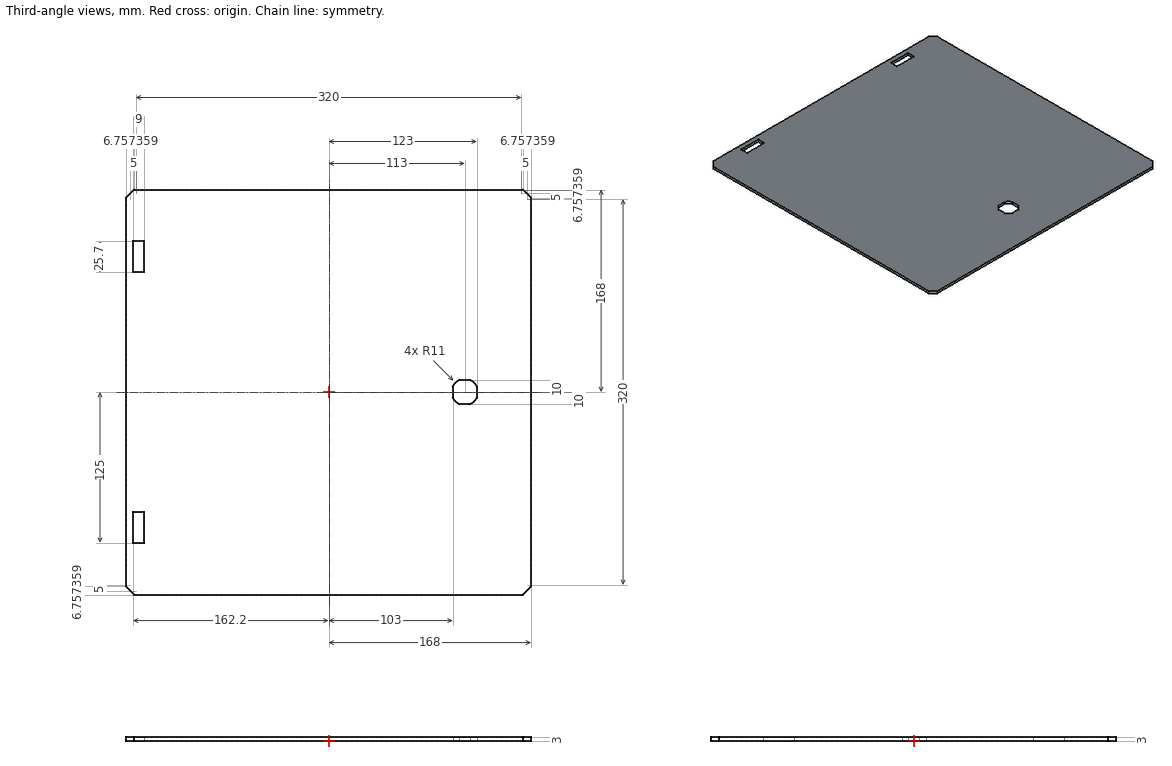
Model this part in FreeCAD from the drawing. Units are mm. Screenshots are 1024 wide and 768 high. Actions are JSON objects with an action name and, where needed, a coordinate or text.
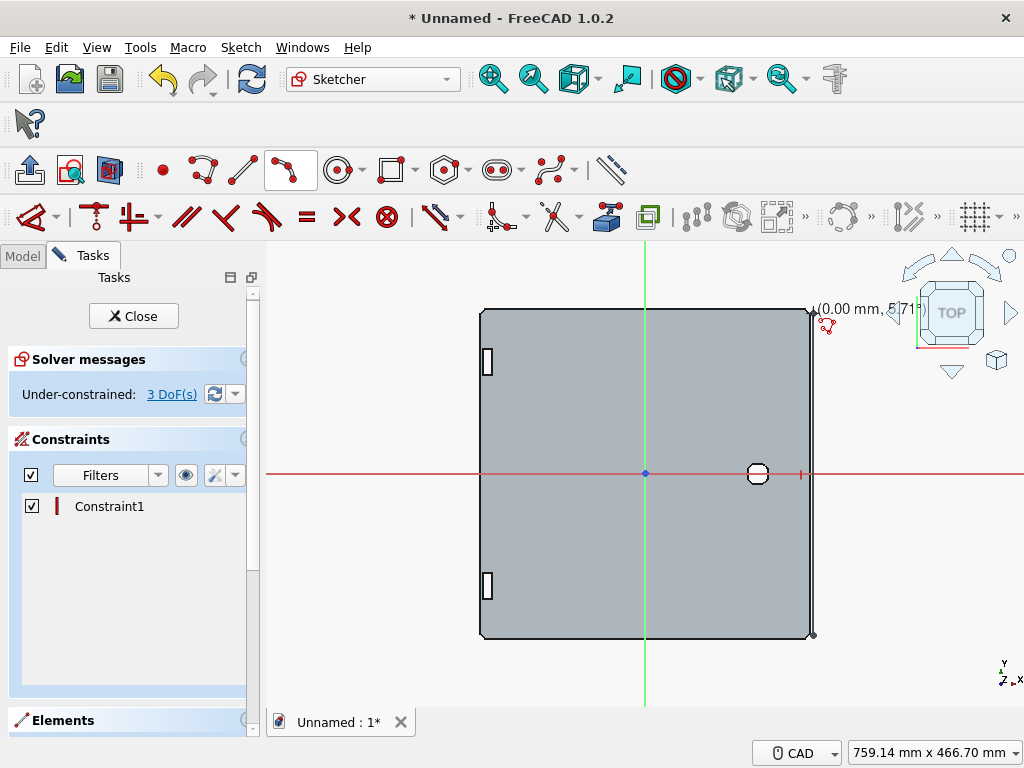
{"action": "scroll", "coordinate": [806, 306], "scroll_direction": "up", "scroll_amount": 3}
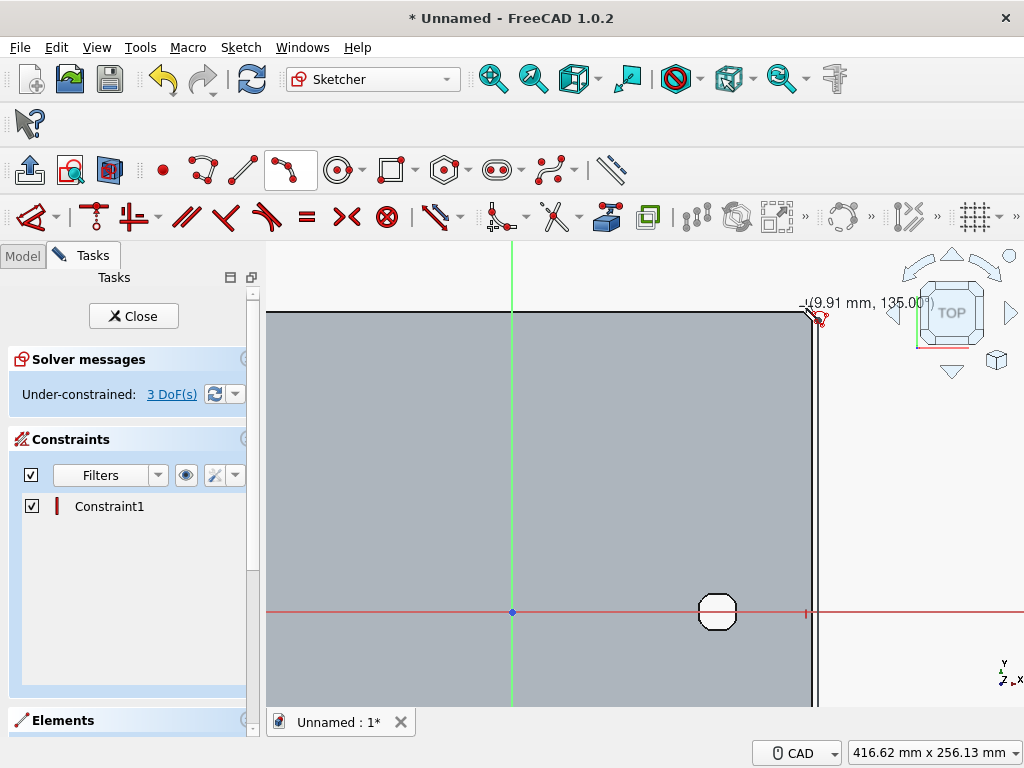
{"action": "left_click", "coordinate": [805, 306]}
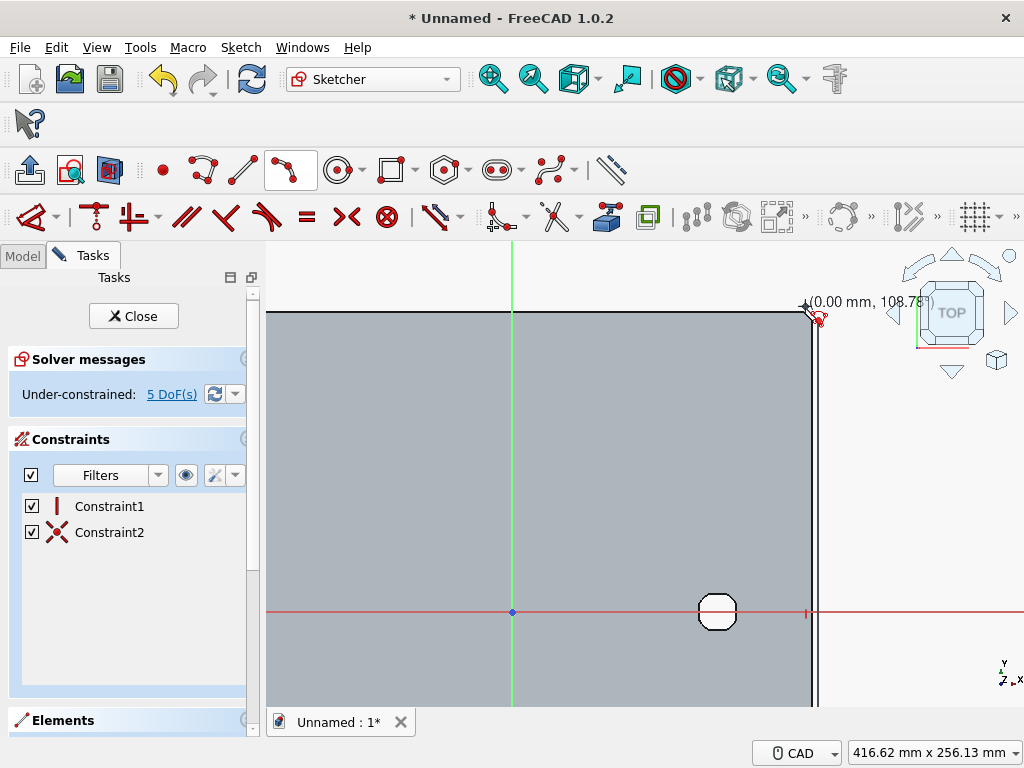
{"action": "scroll", "coordinate": [629, 361], "scroll_direction": "down", "scroll_amount": 4}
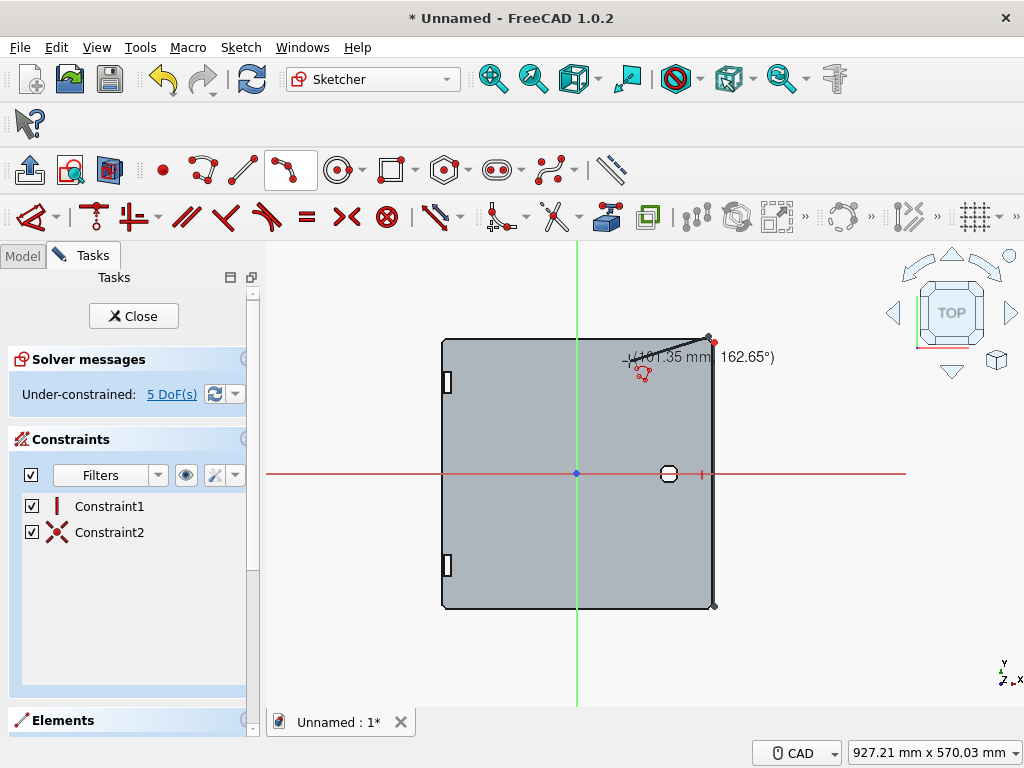
{"action": "left_click", "coordinate": [445, 336]}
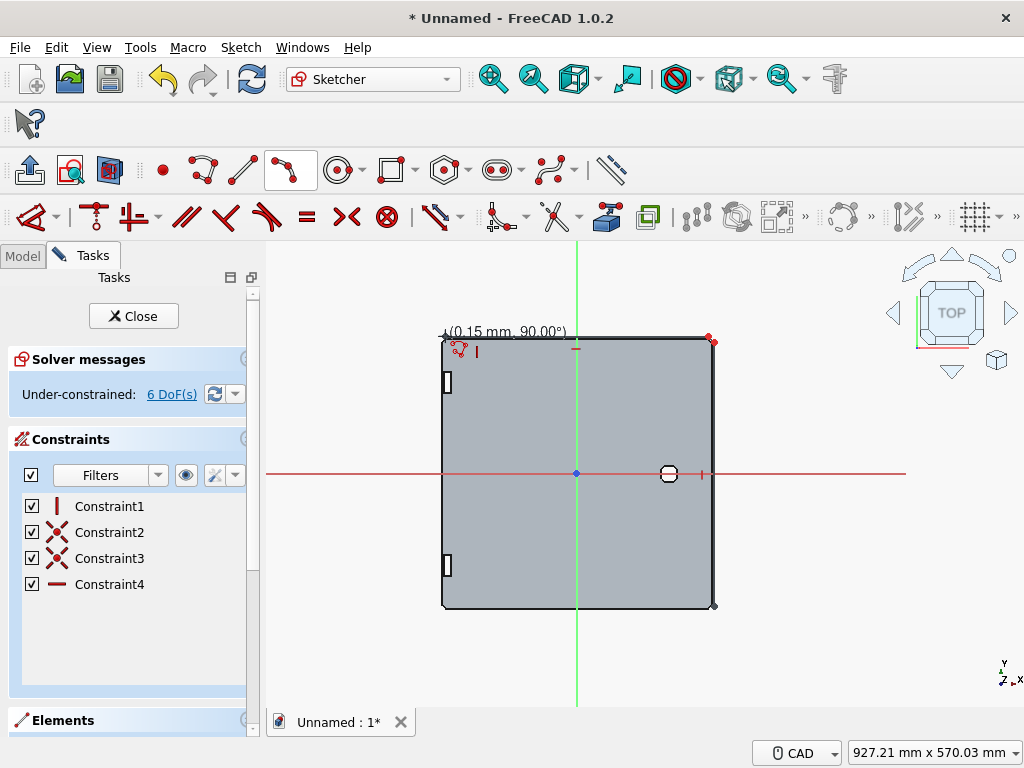
{"action": "scroll", "coordinate": [439, 342], "scroll_direction": "up", "scroll_amount": 4}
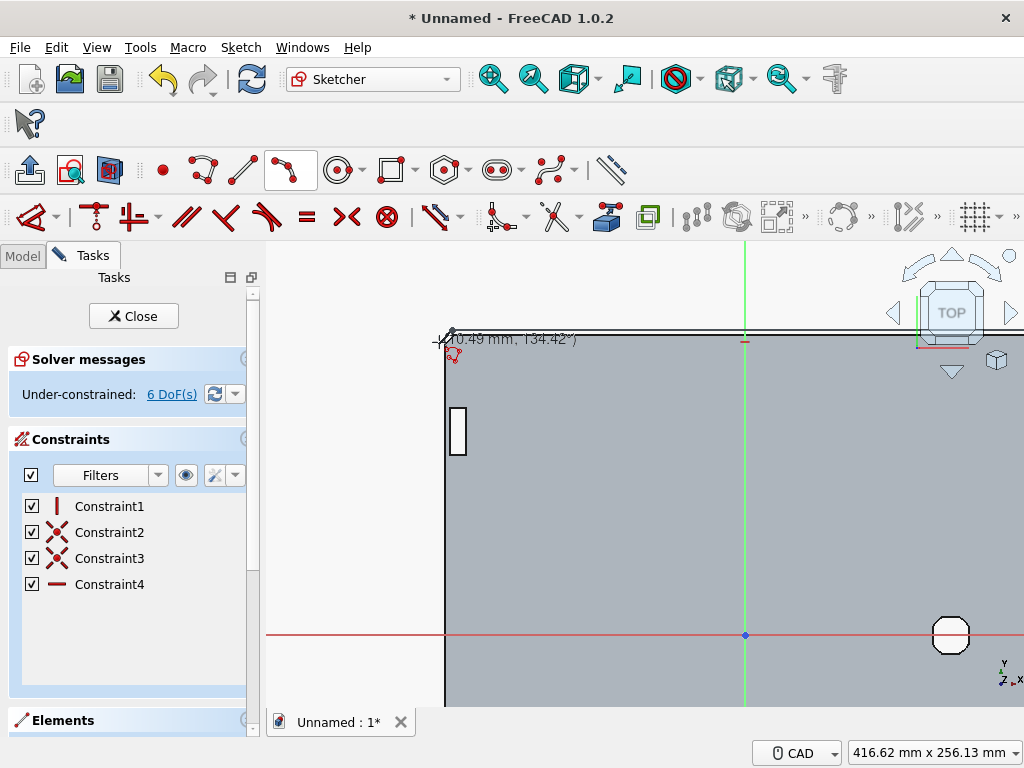
{"action": "left_click", "coordinate": [440, 342]}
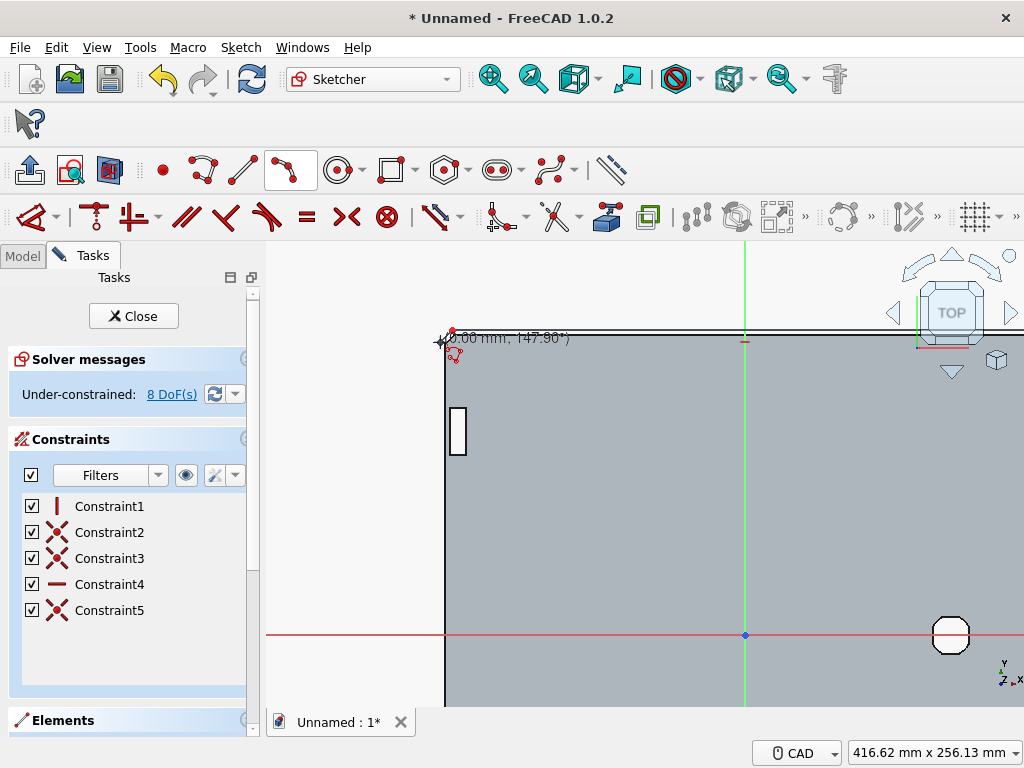
{"action": "scroll", "coordinate": [439, 342], "scroll_direction": "down", "scroll_amount": 4}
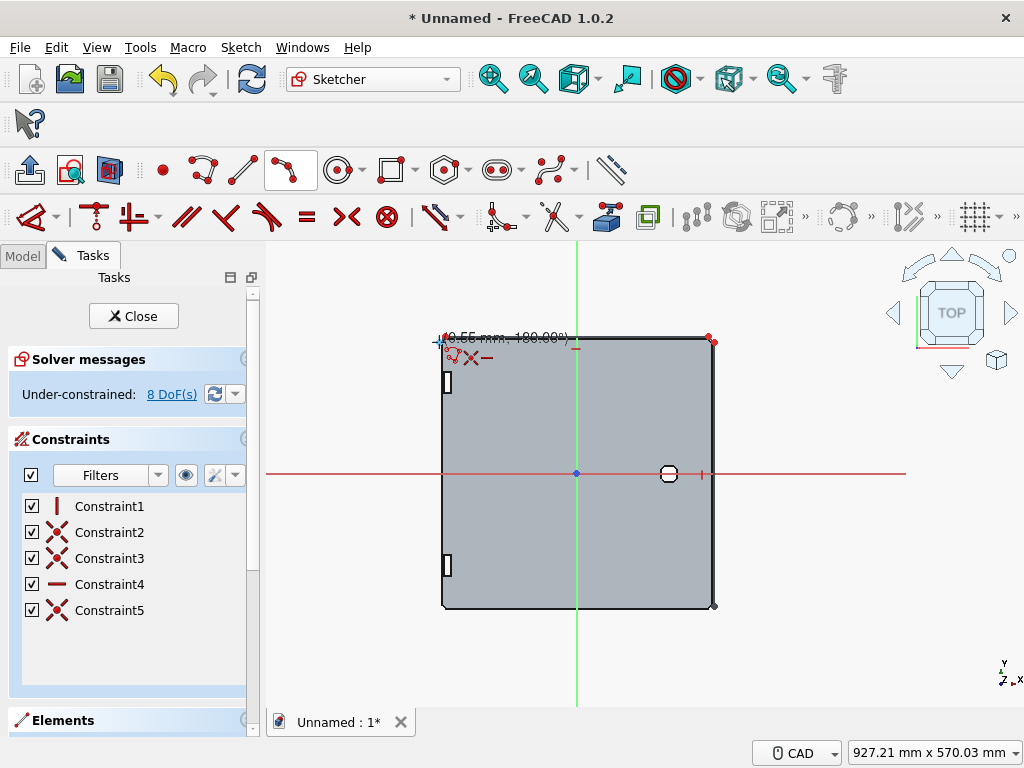
{"action": "left_click", "coordinate": [440, 606]}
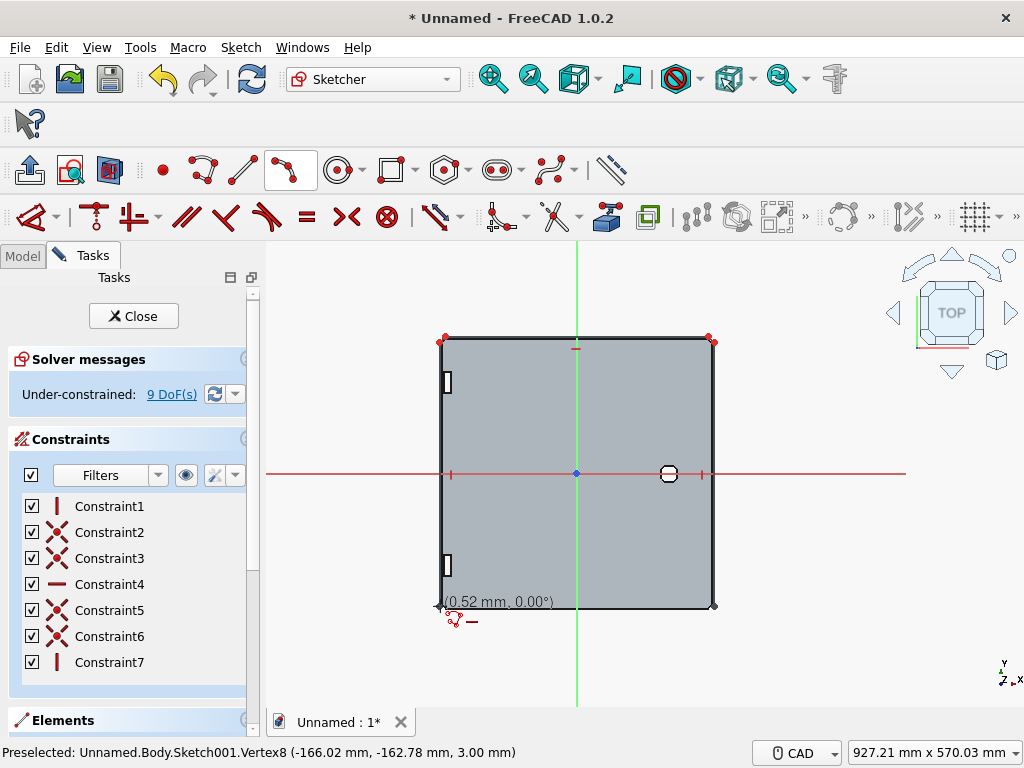
{"action": "scroll", "coordinate": [445, 611], "scroll_direction": "up", "scroll_amount": 4}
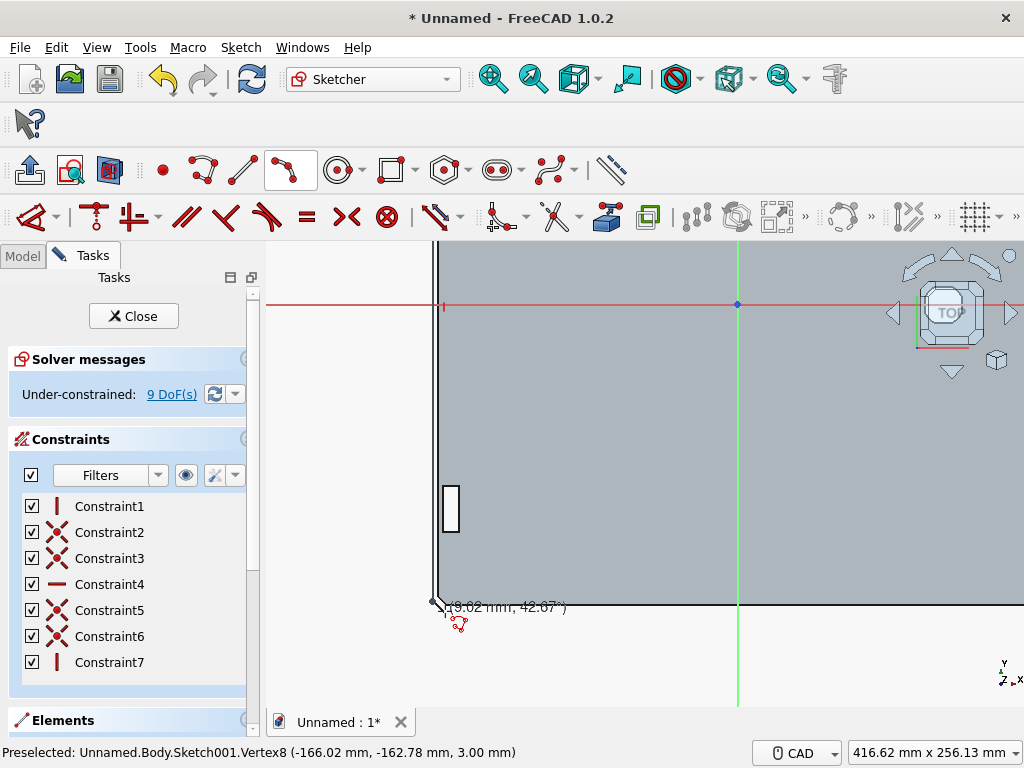
{"action": "left_click", "coordinate": [444, 611]}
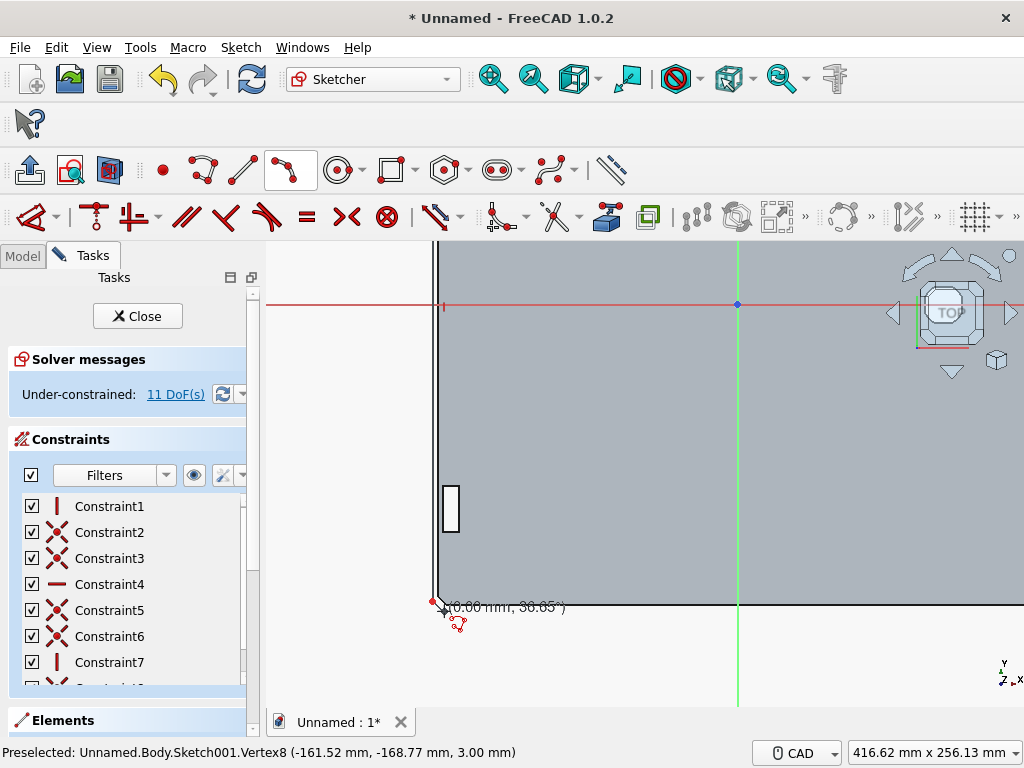
{"action": "scroll", "coordinate": [445, 612], "scroll_direction": "down", "scroll_amount": 4}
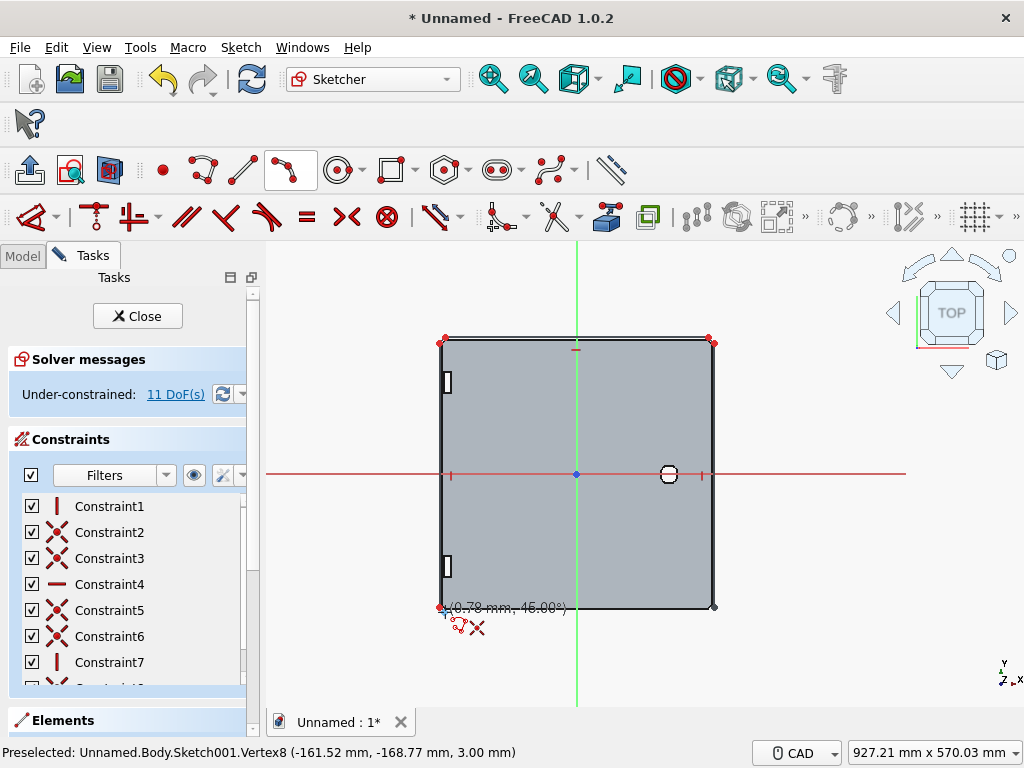
{"action": "scroll", "coordinate": [709, 612], "scroll_direction": "up", "scroll_amount": 4}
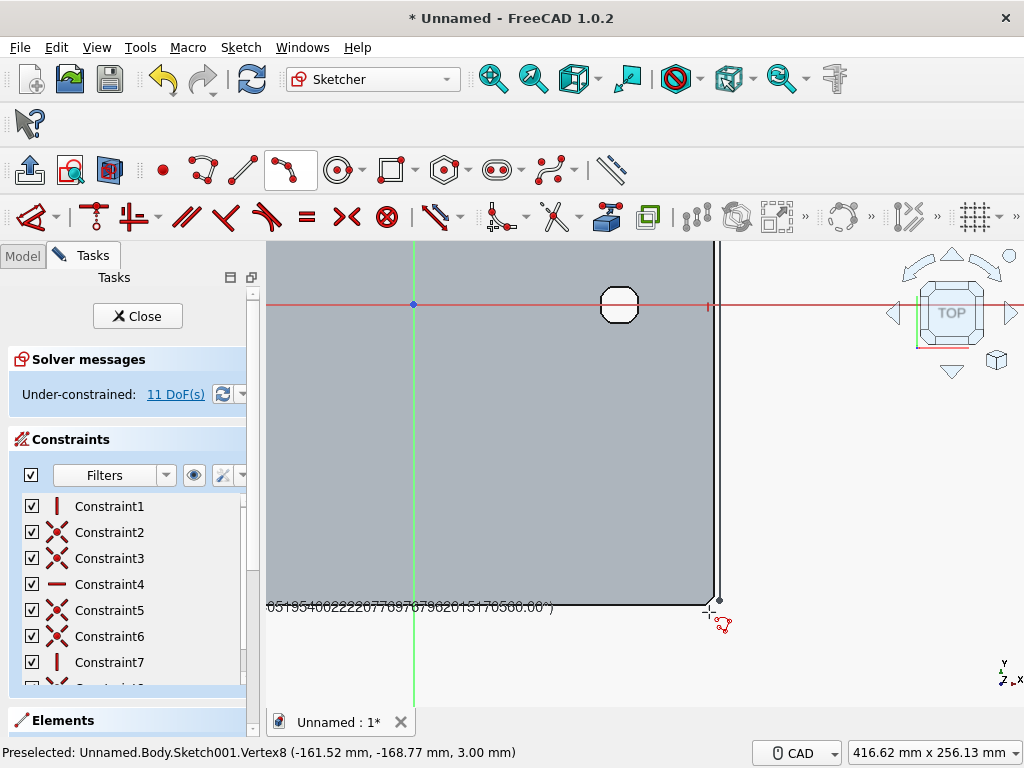
{"action": "left_click", "coordinate": [707, 611]}
{"action": "left_click", "coordinate": [720, 600]}